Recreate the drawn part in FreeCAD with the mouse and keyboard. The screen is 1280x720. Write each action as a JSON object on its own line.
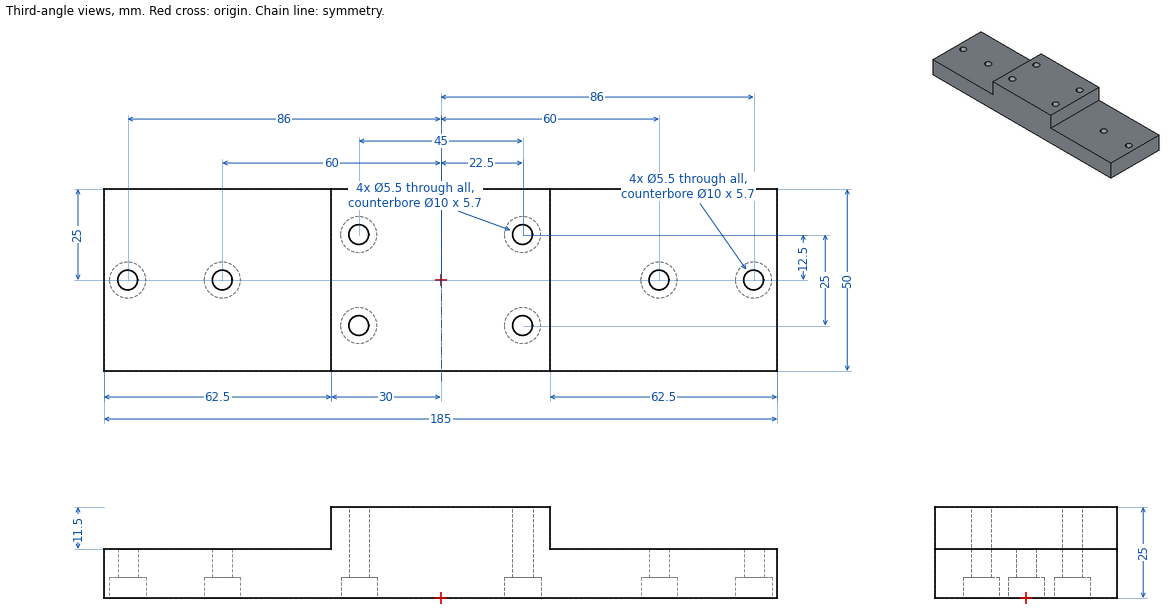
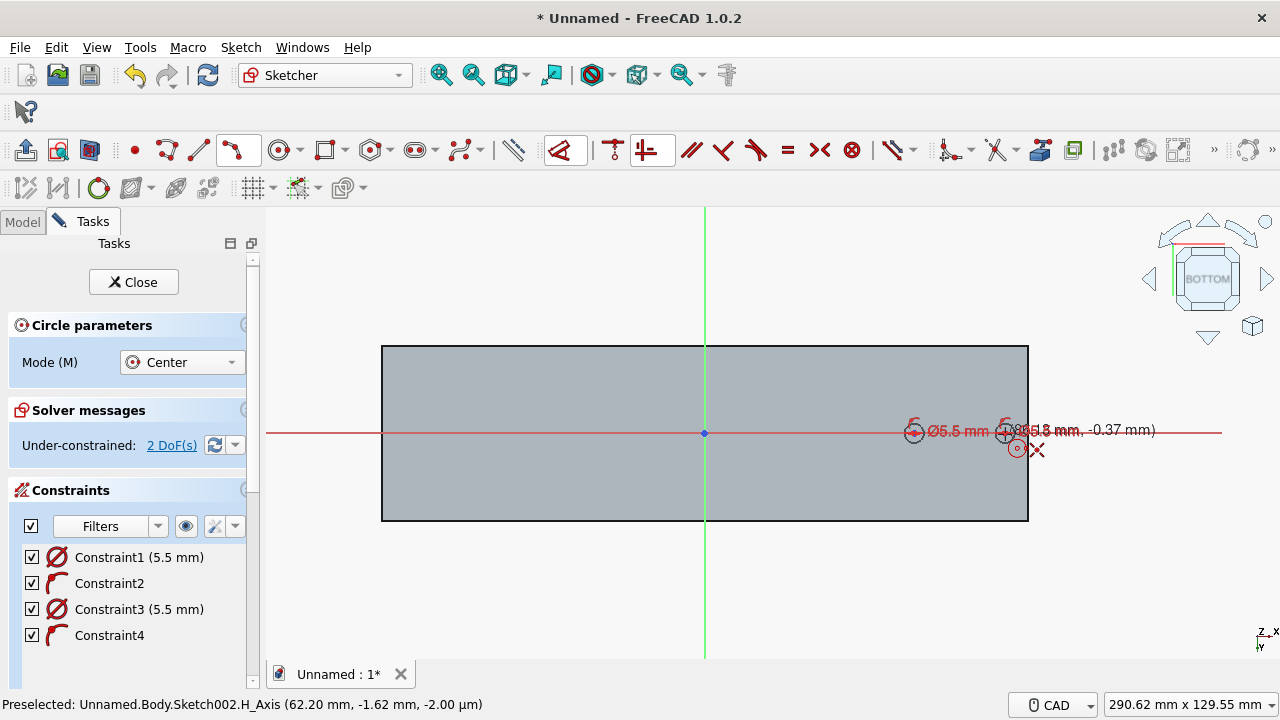
{"action": "scroll", "coordinate": [496, 433], "scroll_direction": "up", "scroll_amount": 5}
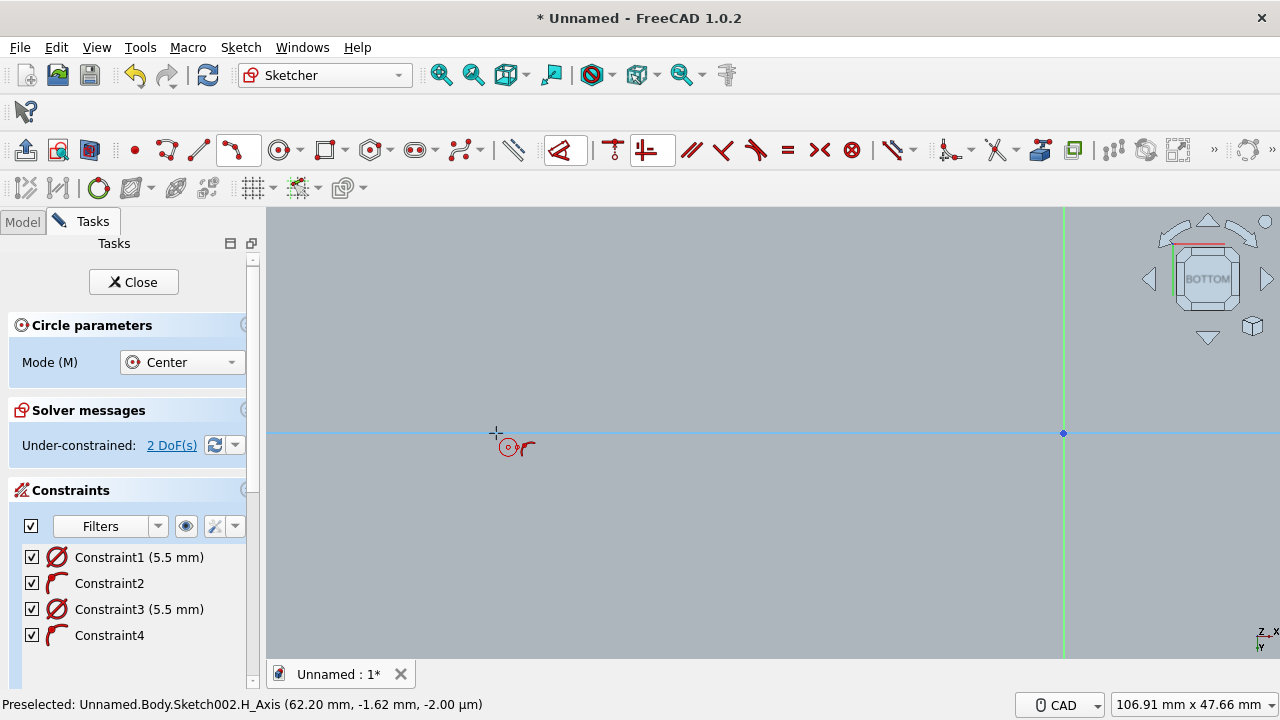
{"action": "left_click", "coordinate": [495, 433]}
{"action": "mouse_move", "coordinate": [513, 415]}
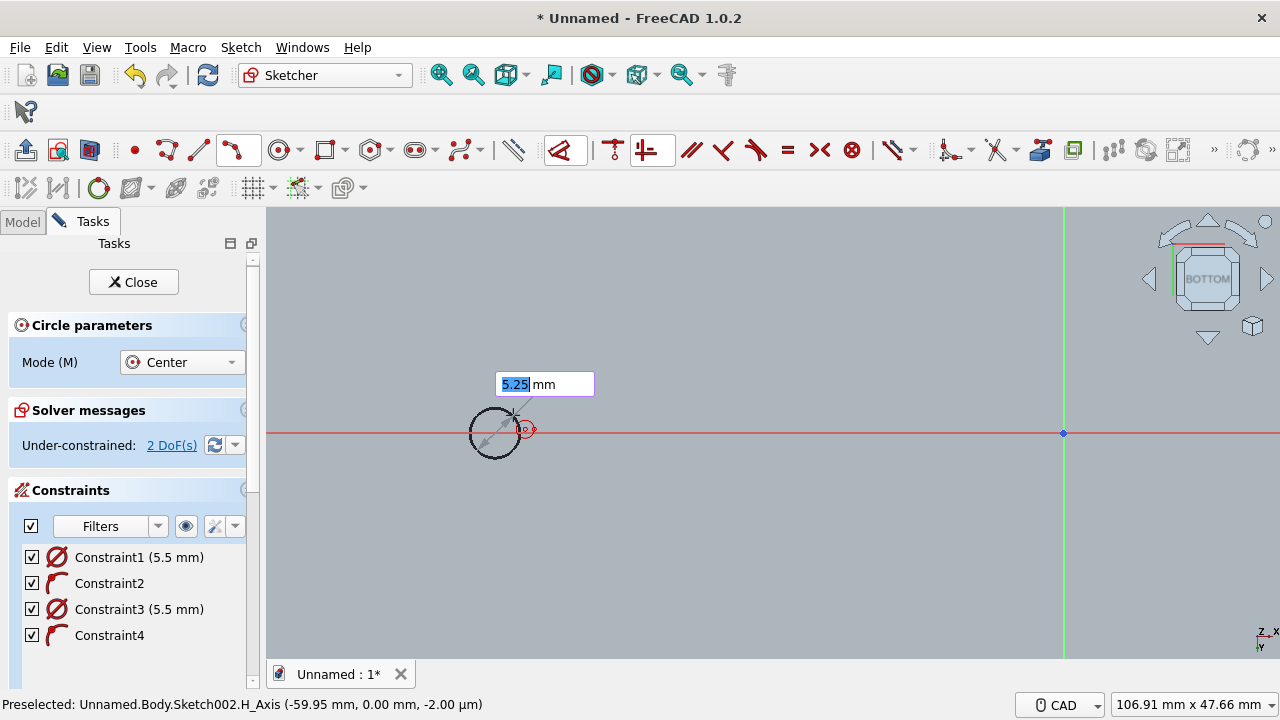
{"action": "type", "text": "5.5"}
{"action": "key", "text": "Return"}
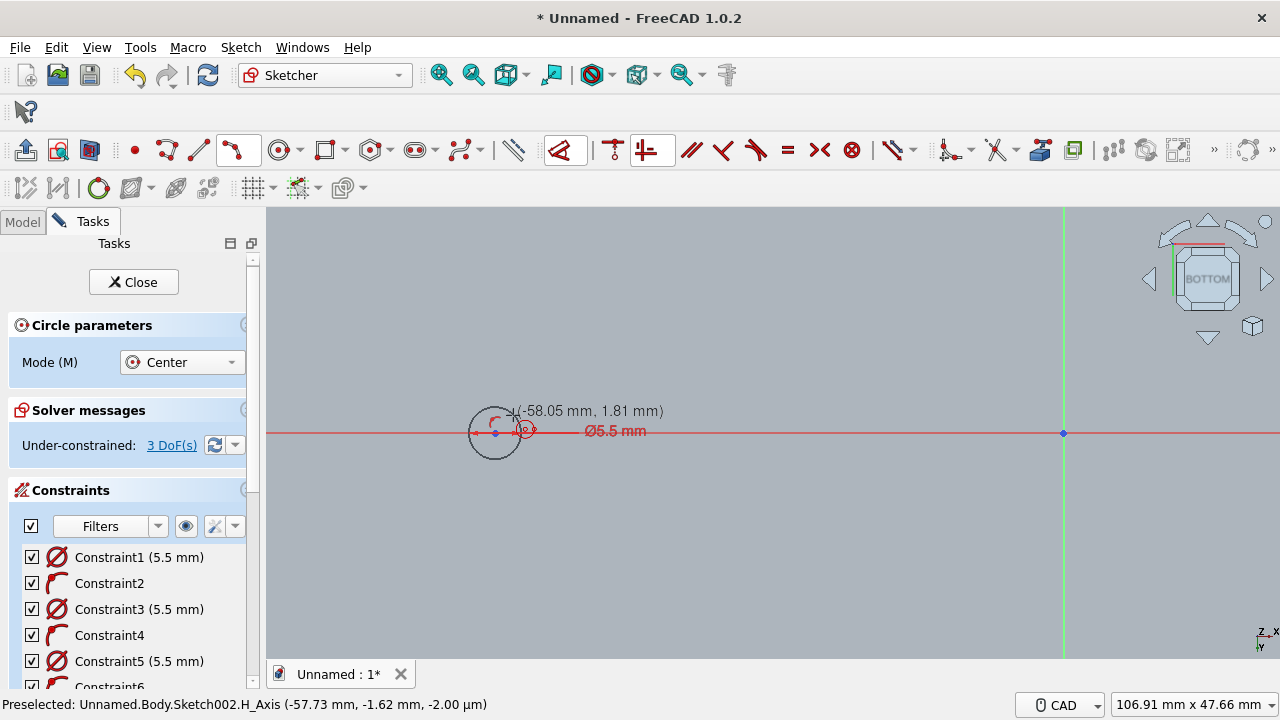
{"action": "scroll", "coordinate": [496, 433], "scroll_direction": "down", "scroll_amount": 5}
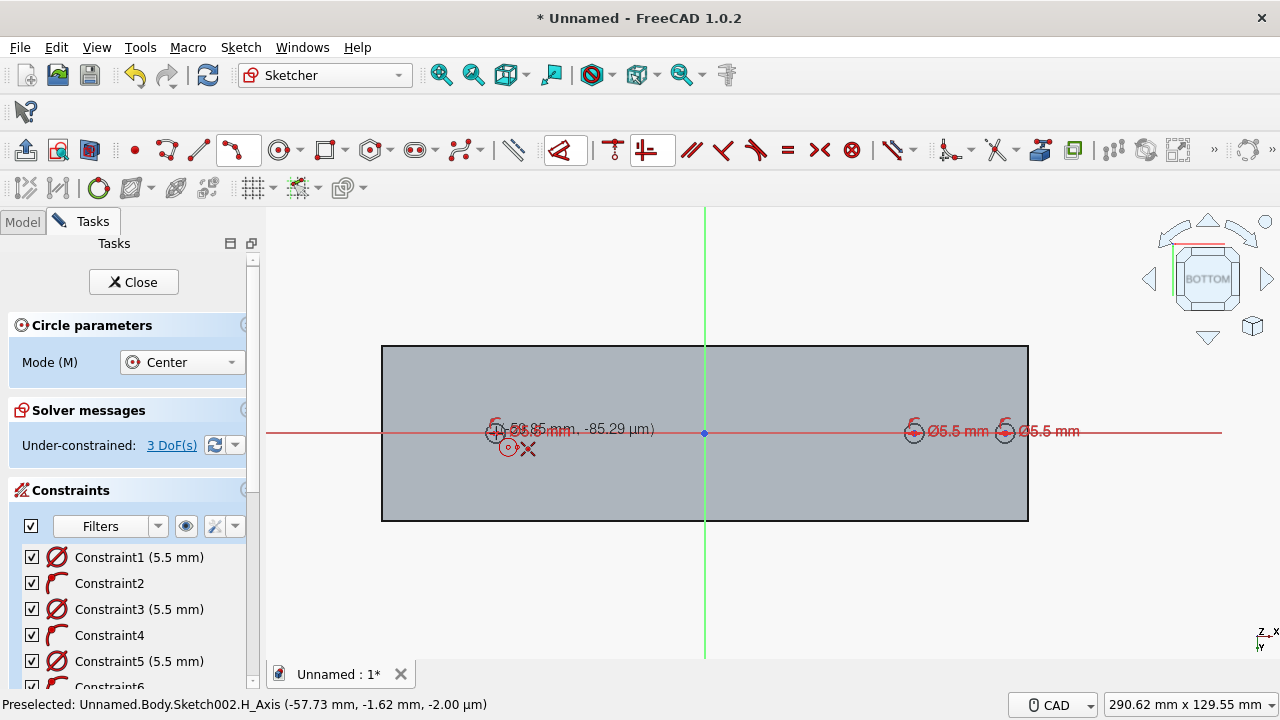
{"action": "scroll", "coordinate": [405, 433], "scroll_direction": "up", "scroll_amount": 5}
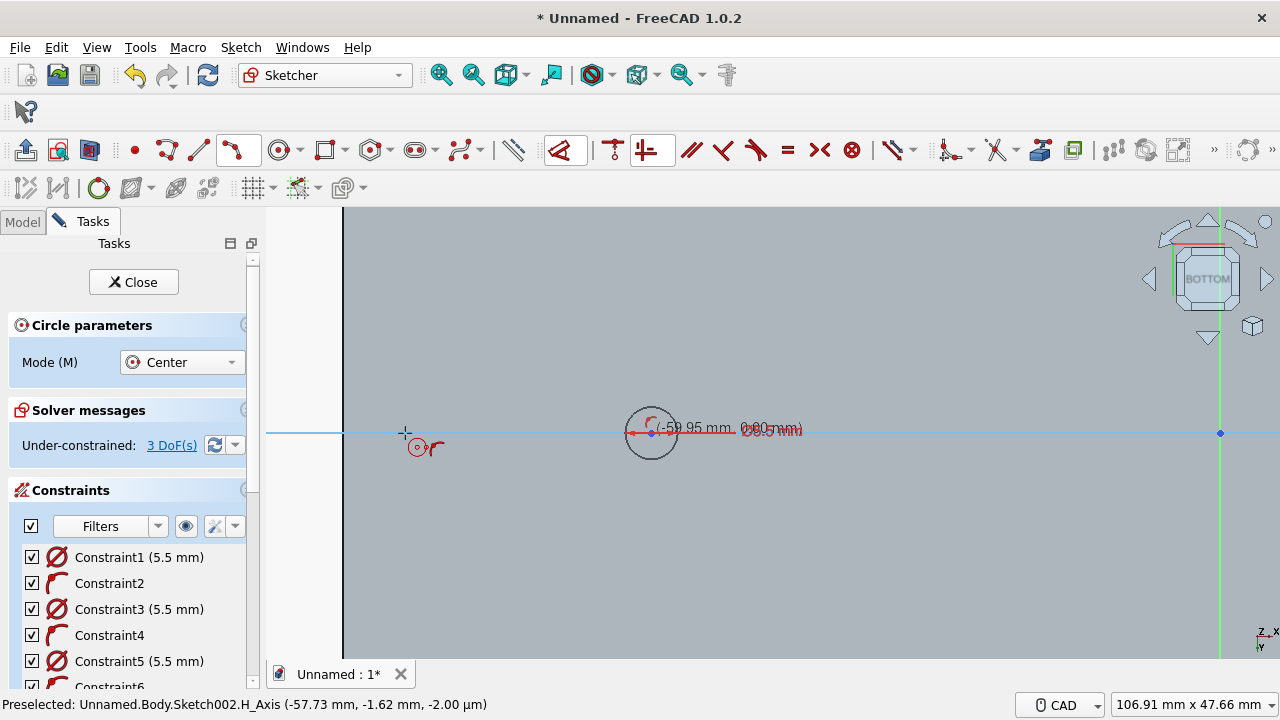
{"action": "left_click", "coordinate": [404, 433]}
{"action": "mouse_move", "coordinate": [423, 415]}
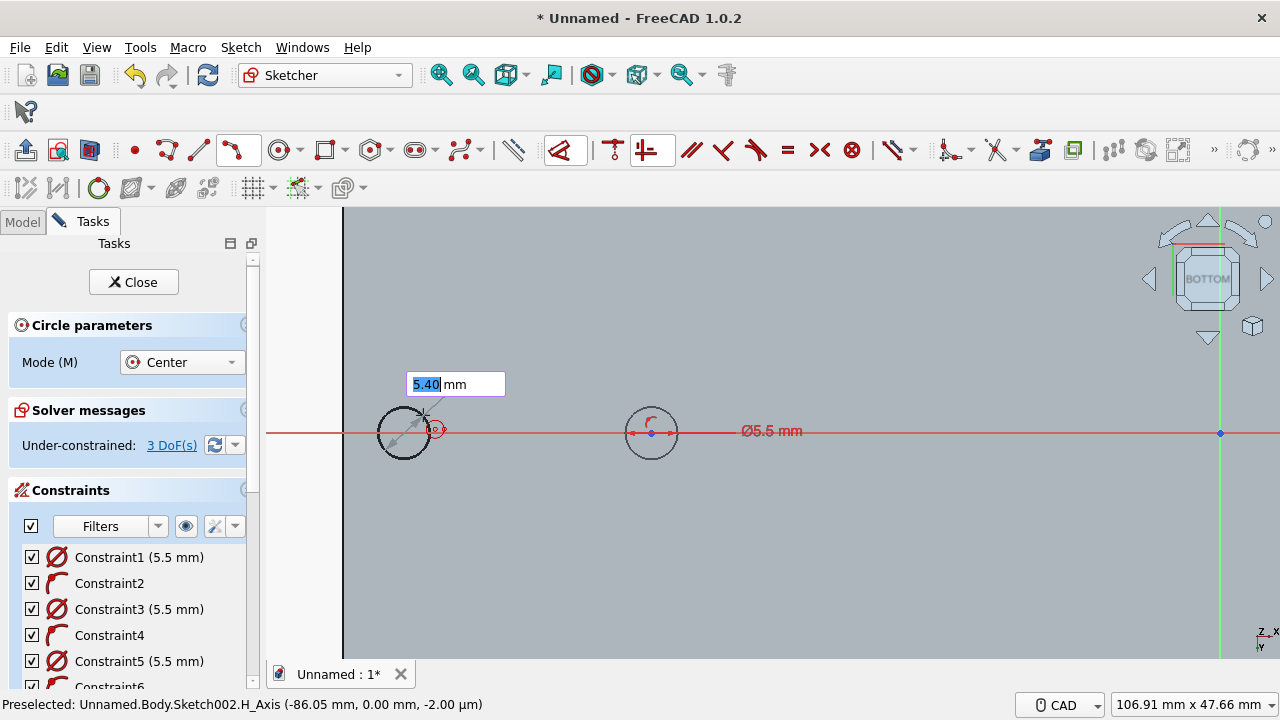
{"action": "type", "text": "5.5"}
{"action": "key", "text": "Return"}
{"action": "key", "text": "Escape"}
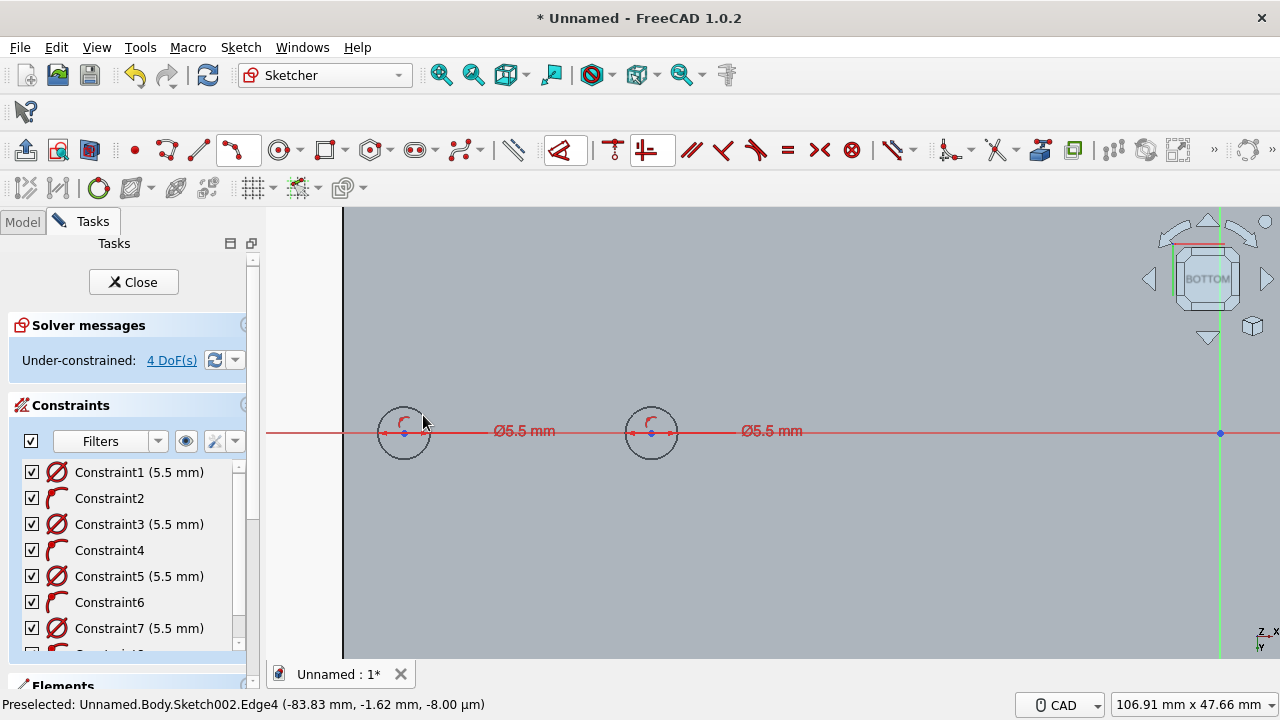
{"action": "left_click", "coordinate": [560, 150]}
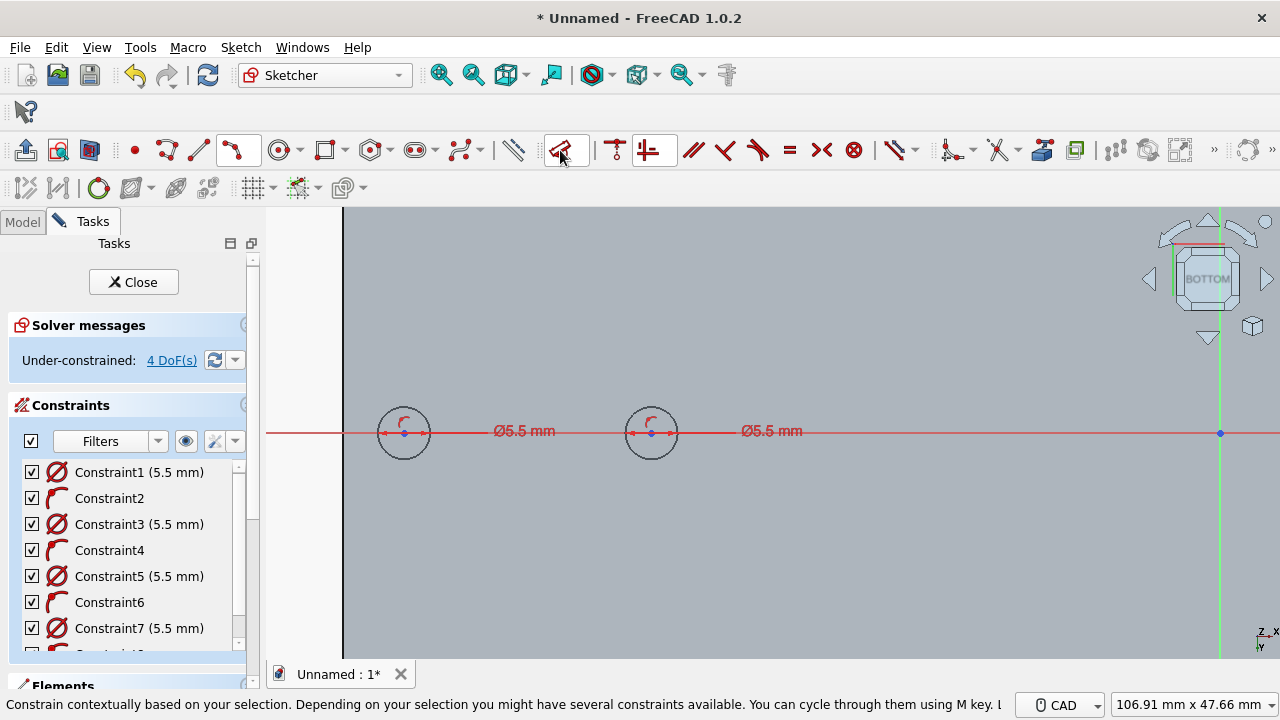
{"action": "scroll", "coordinate": [404, 433], "scroll_direction": "down", "scroll_amount": 5}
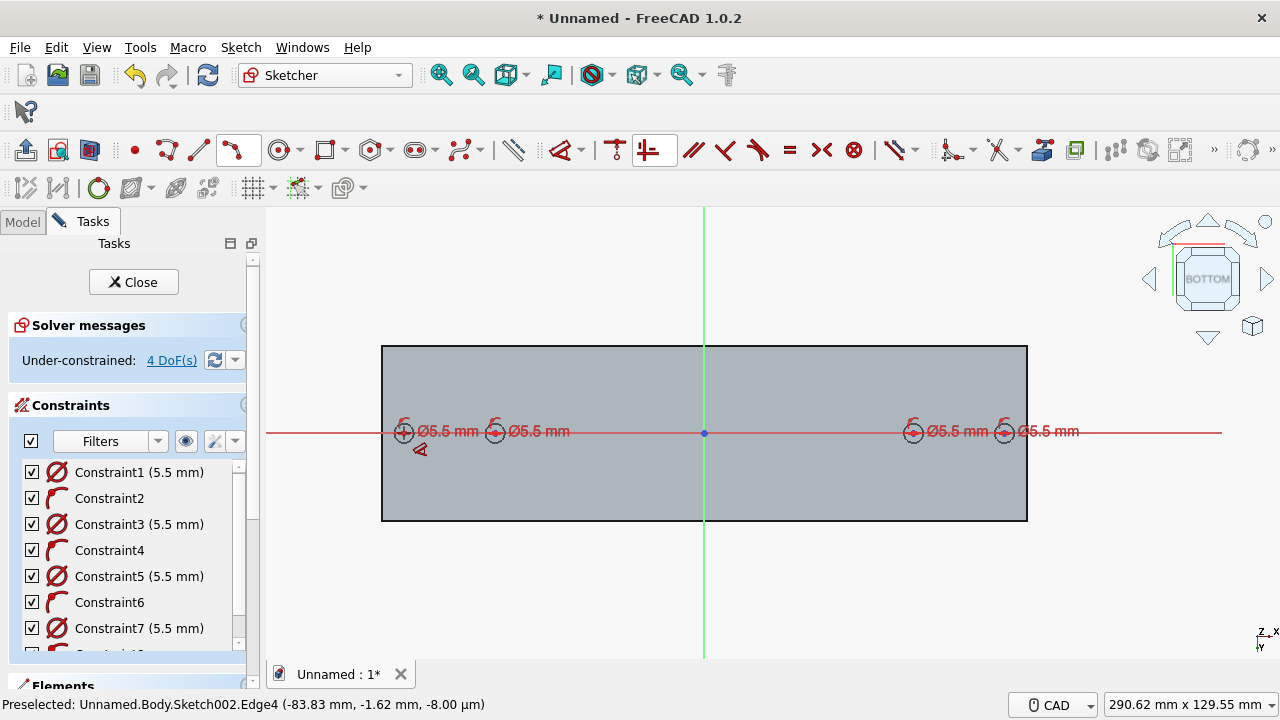
{"action": "left_click", "coordinate": [1004, 433]}
{"action": "left_click", "coordinate": [854, 467]}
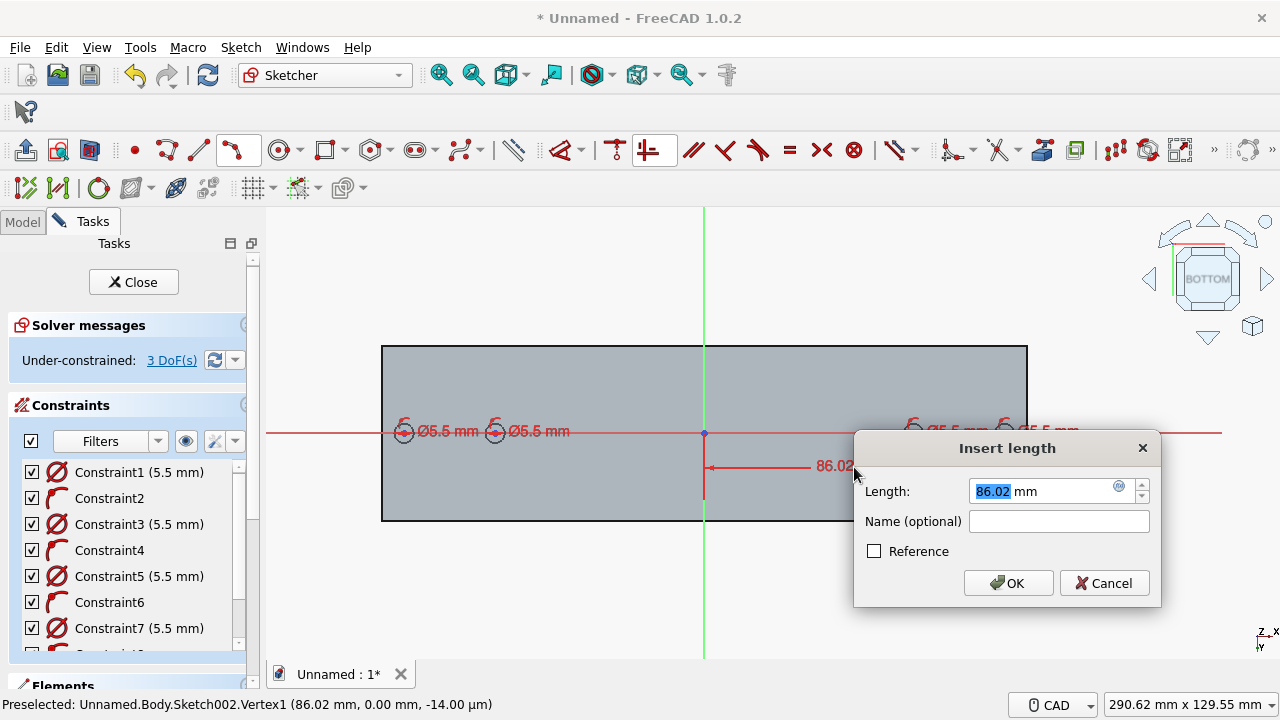
{"action": "type", "text": "86"}
{"action": "key", "text": "Return"}